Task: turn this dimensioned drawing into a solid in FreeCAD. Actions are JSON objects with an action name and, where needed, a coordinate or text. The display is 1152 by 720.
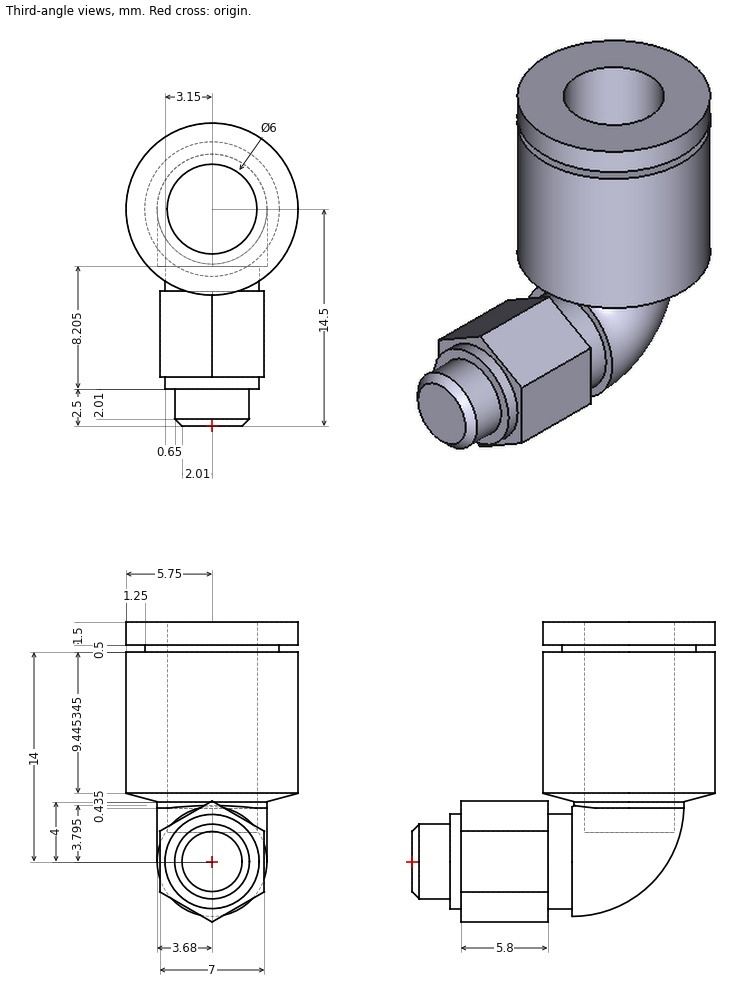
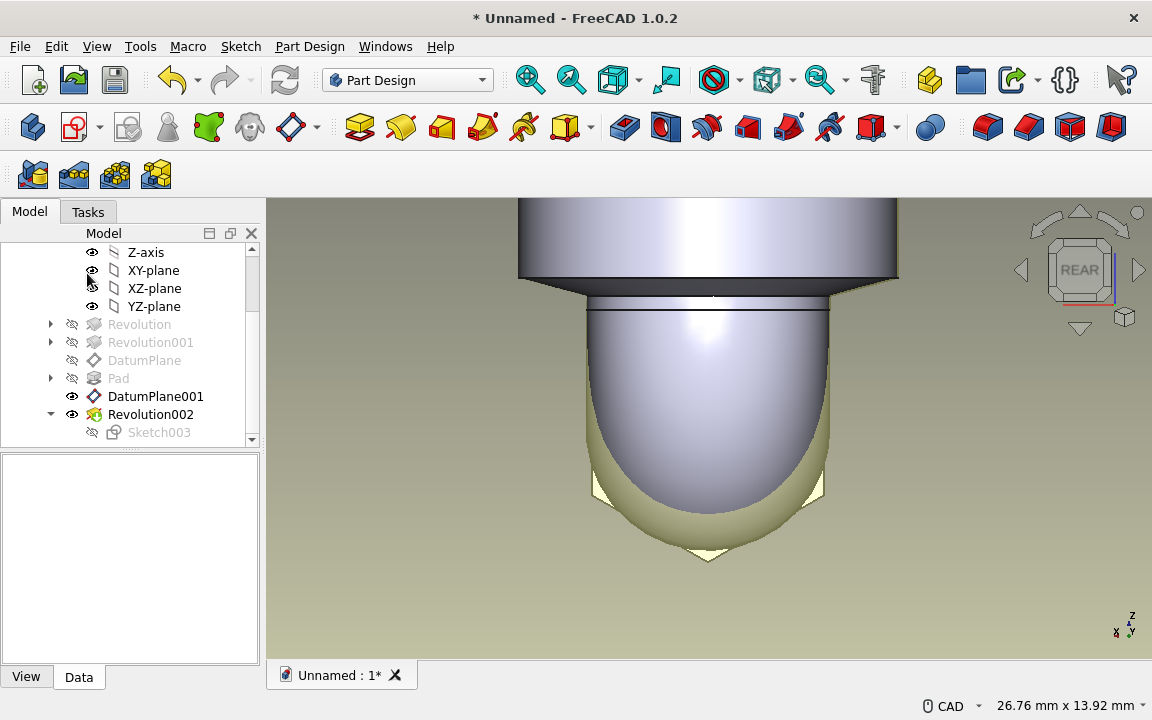
{"action": "left_click", "coordinate": [117, 396]}
{"action": "key", "text": "space"}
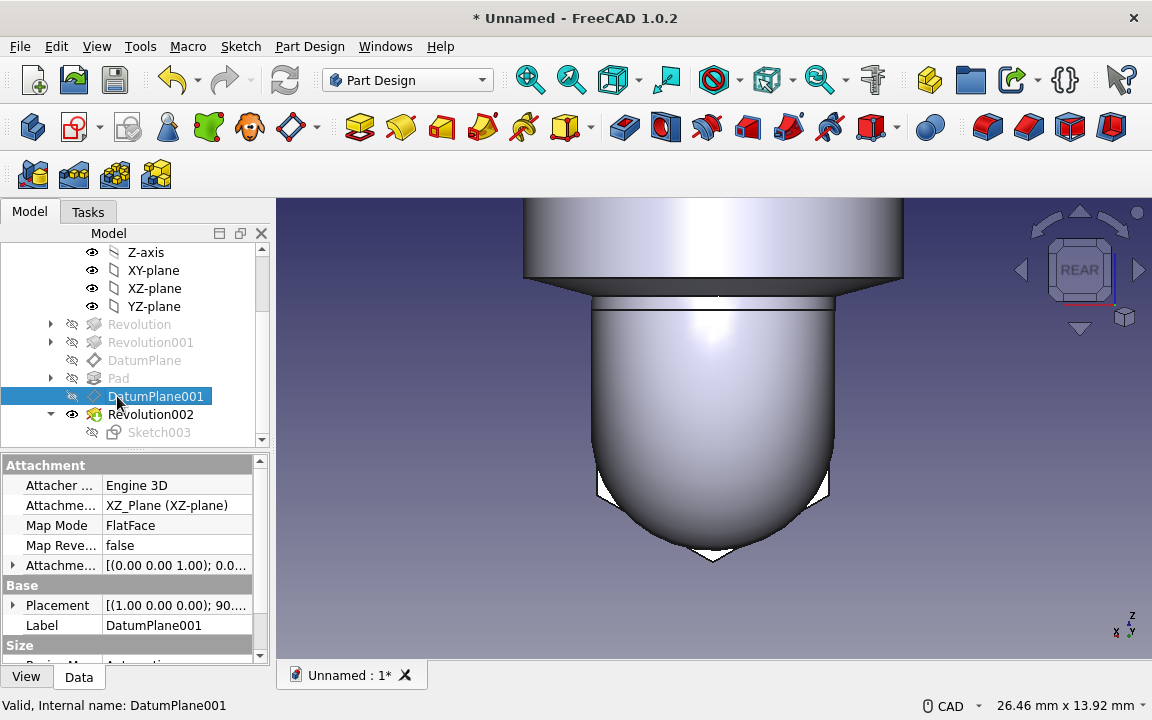
{"action": "left_click", "coordinate": [531, 80]}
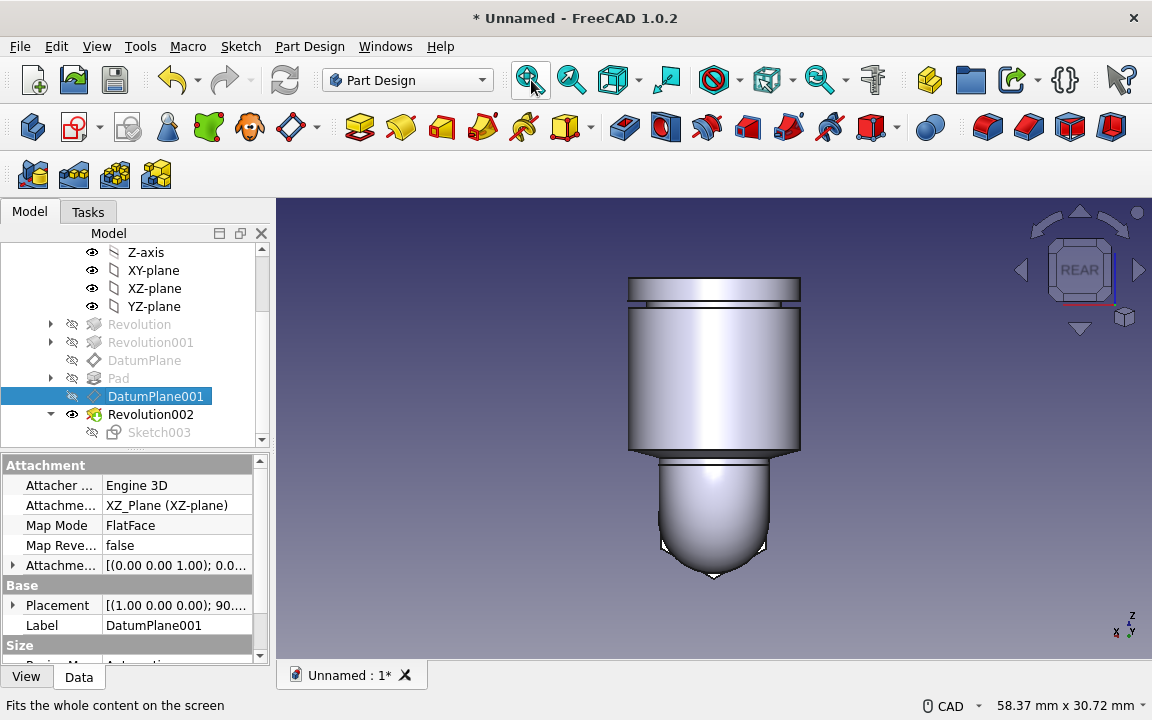
{"action": "key", "text": "0"}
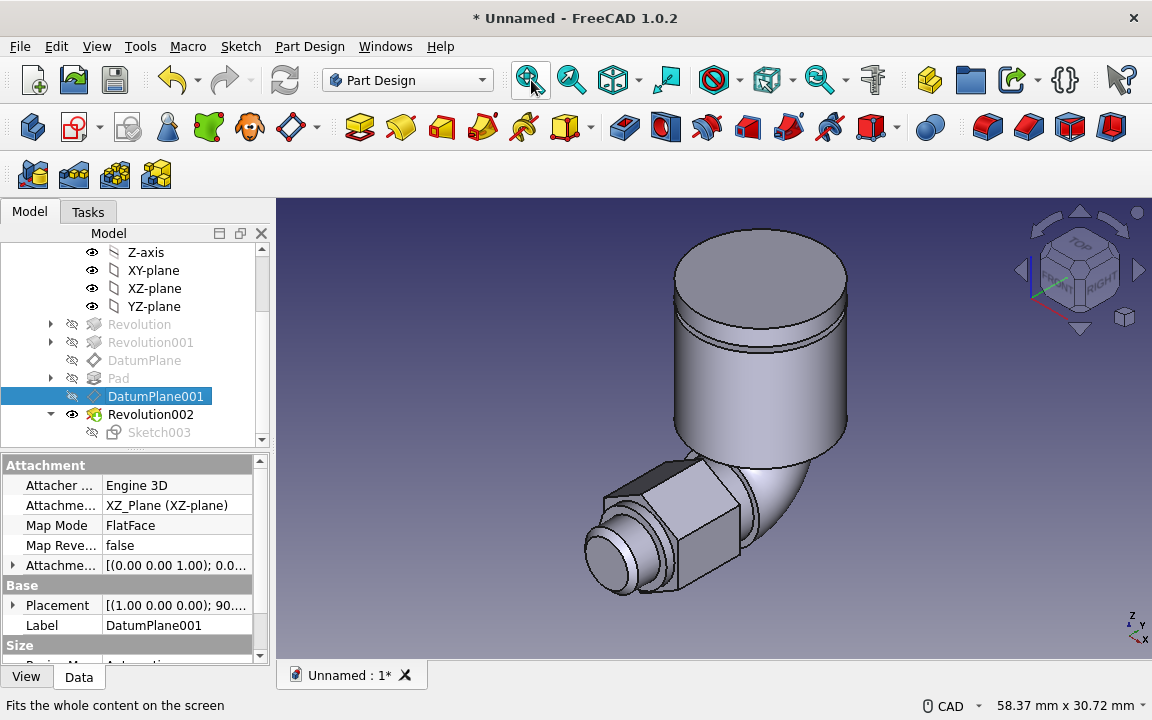
{"action": "left_click", "coordinate": [761, 278]}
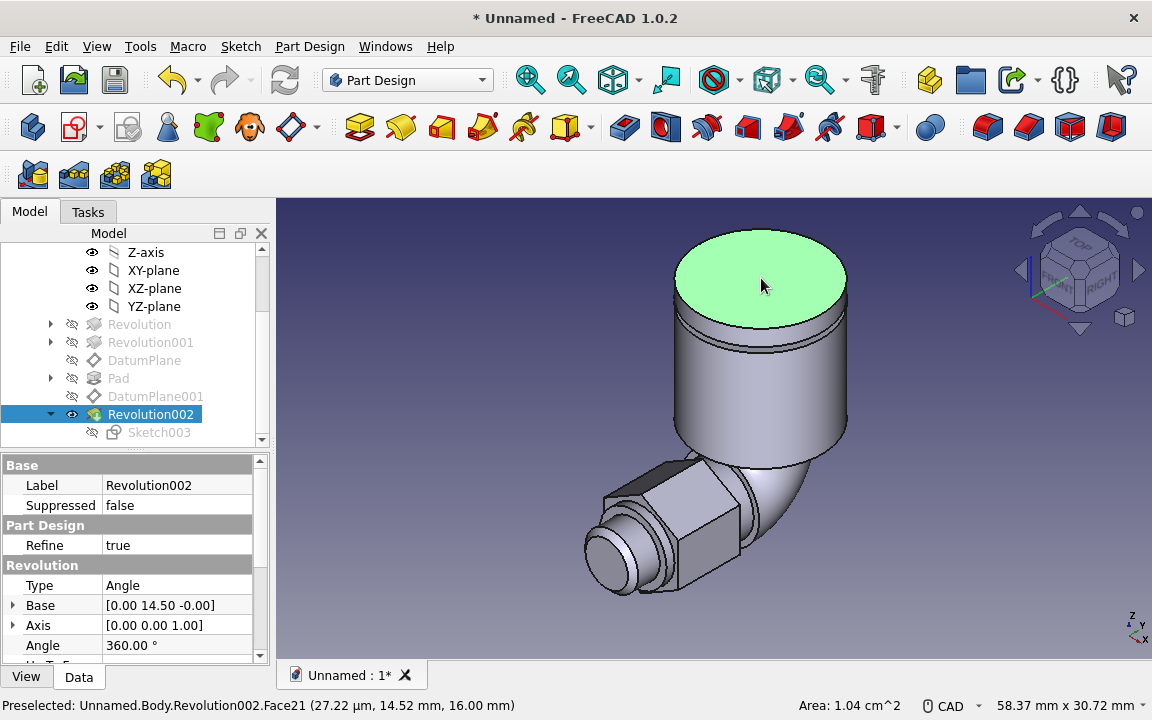
{"action": "left_click", "coordinate": [74, 128]}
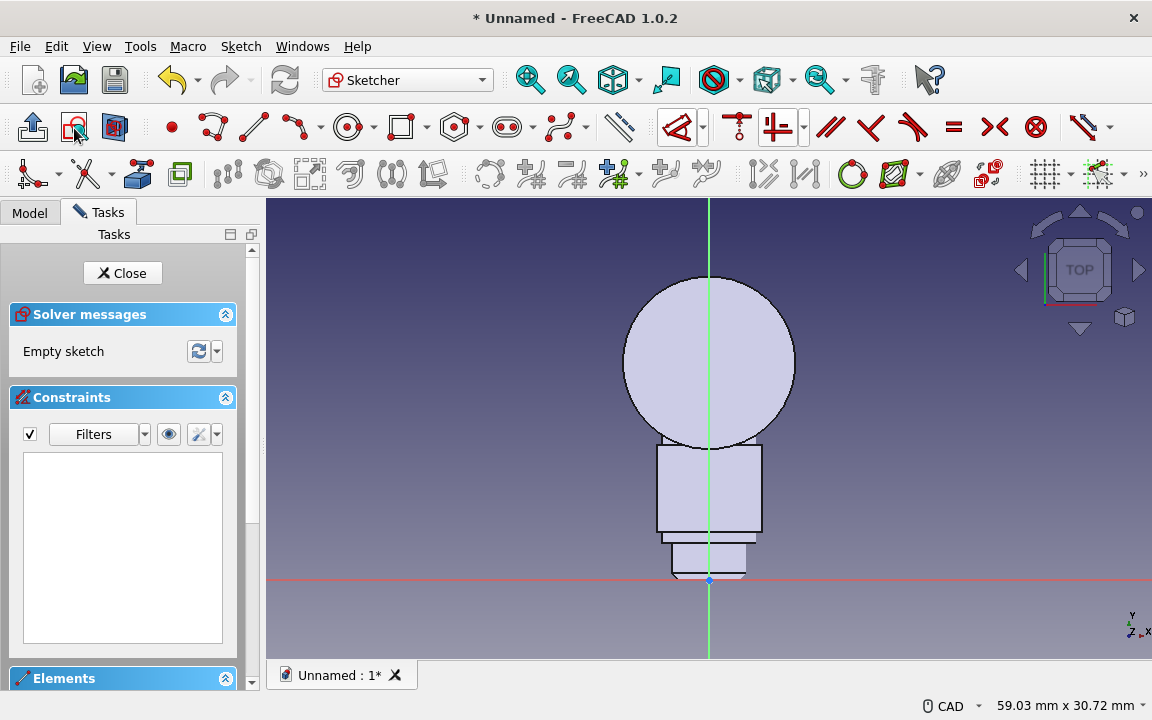
{"action": "scroll", "coordinate": [739, 334], "scroll_direction": "up", "scroll_amount": 6}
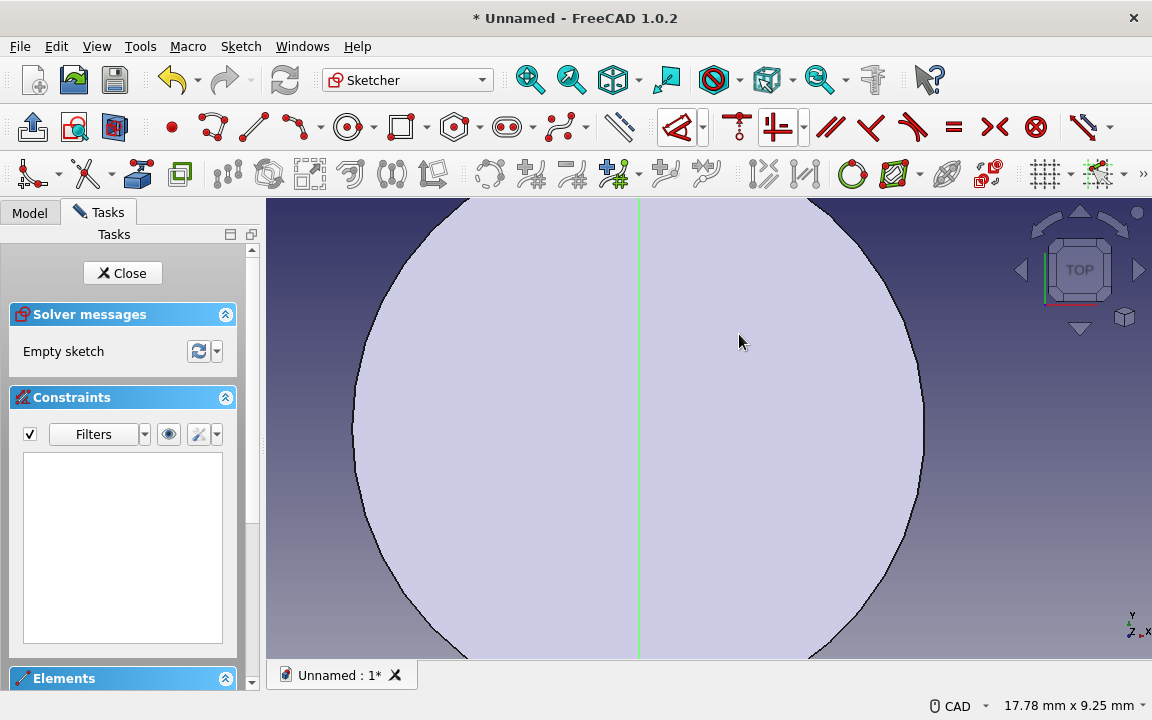
{"action": "left_click", "coordinate": [348, 128]}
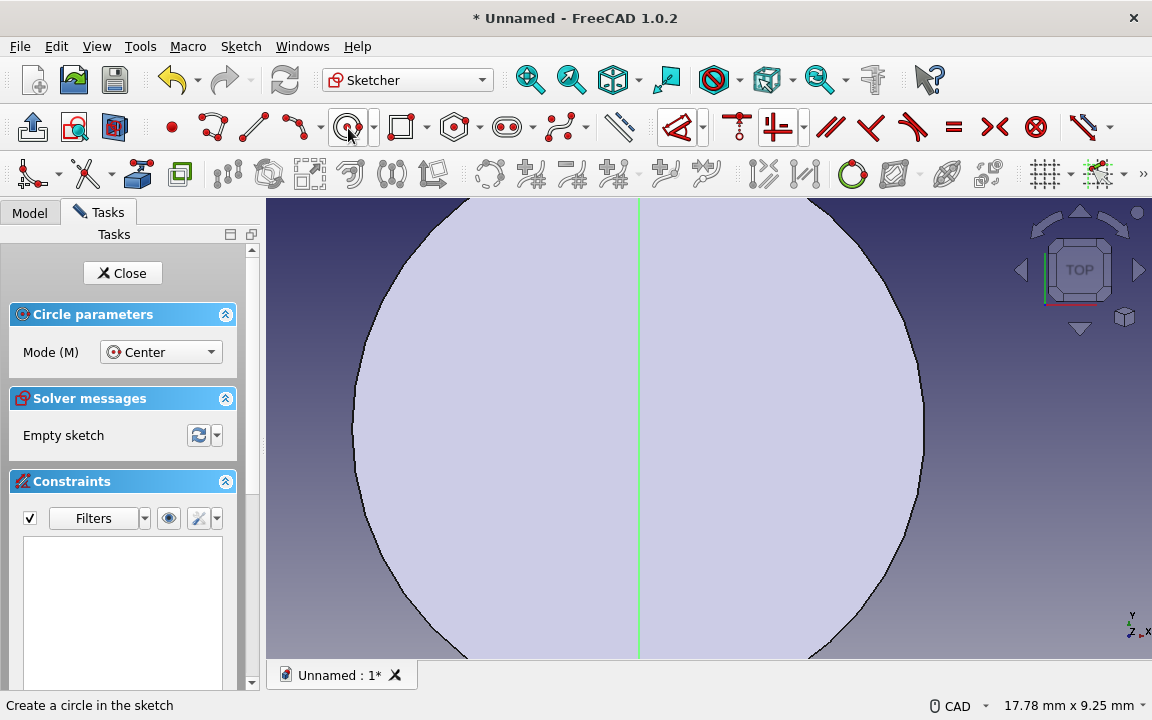
{"action": "left_click", "coordinate": [639, 429]}
{"action": "left_click", "coordinate": [744, 323]}
{"action": "key", "text": "Escape"}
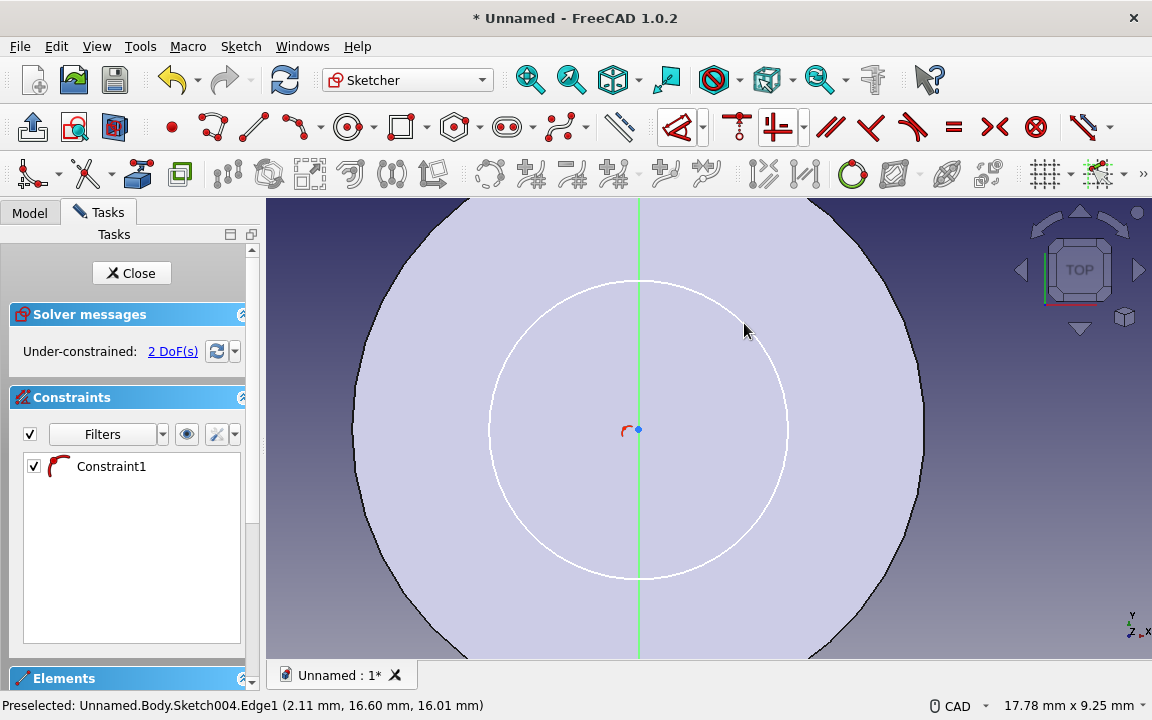
{"action": "left_click", "coordinate": [744, 324]}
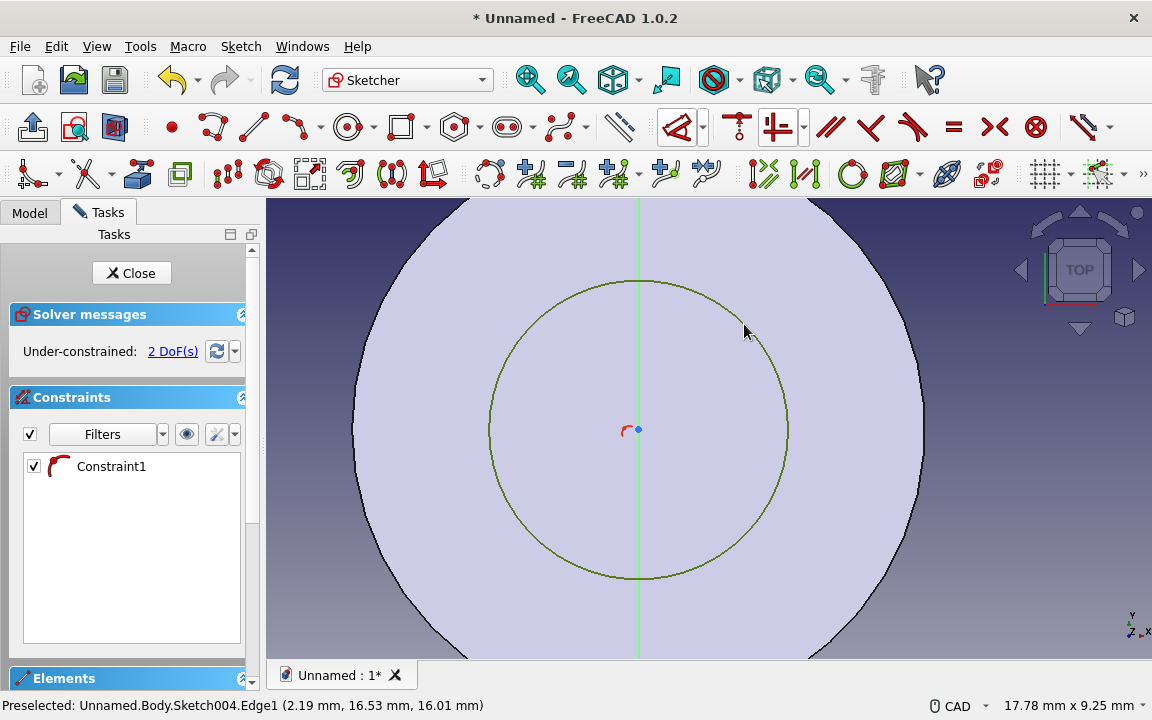
{"action": "key", "text": "k o"}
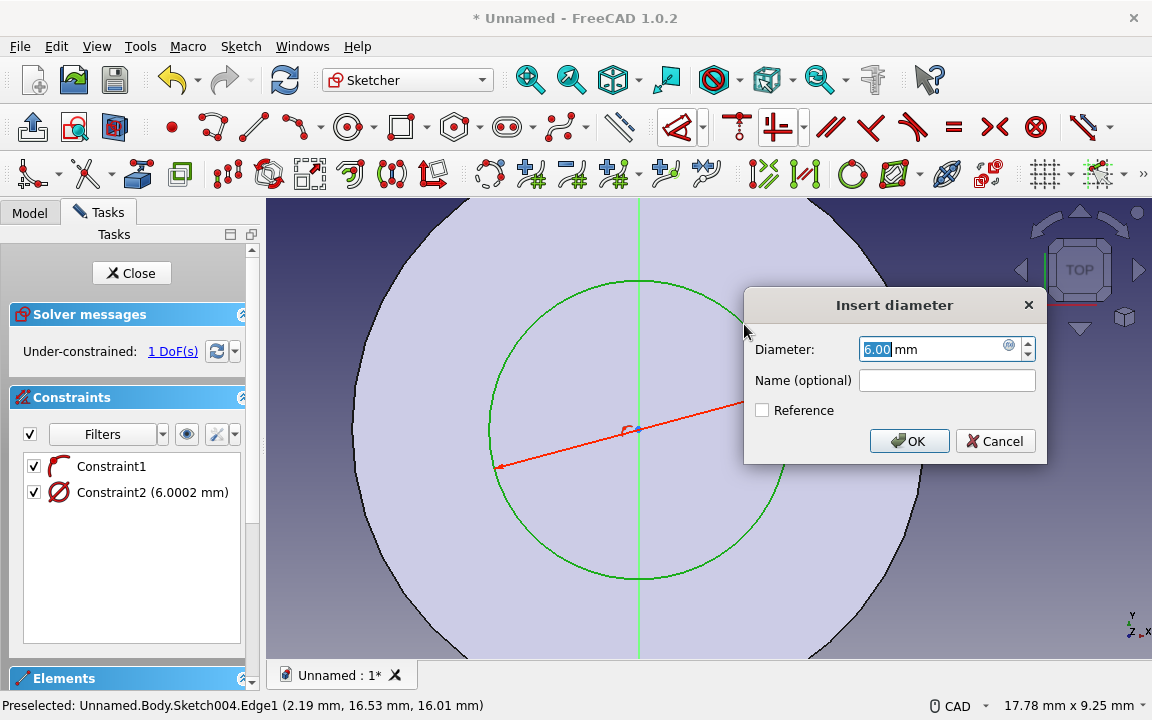
{"action": "type", "text": "6"}
{"action": "key", "text": "Return"}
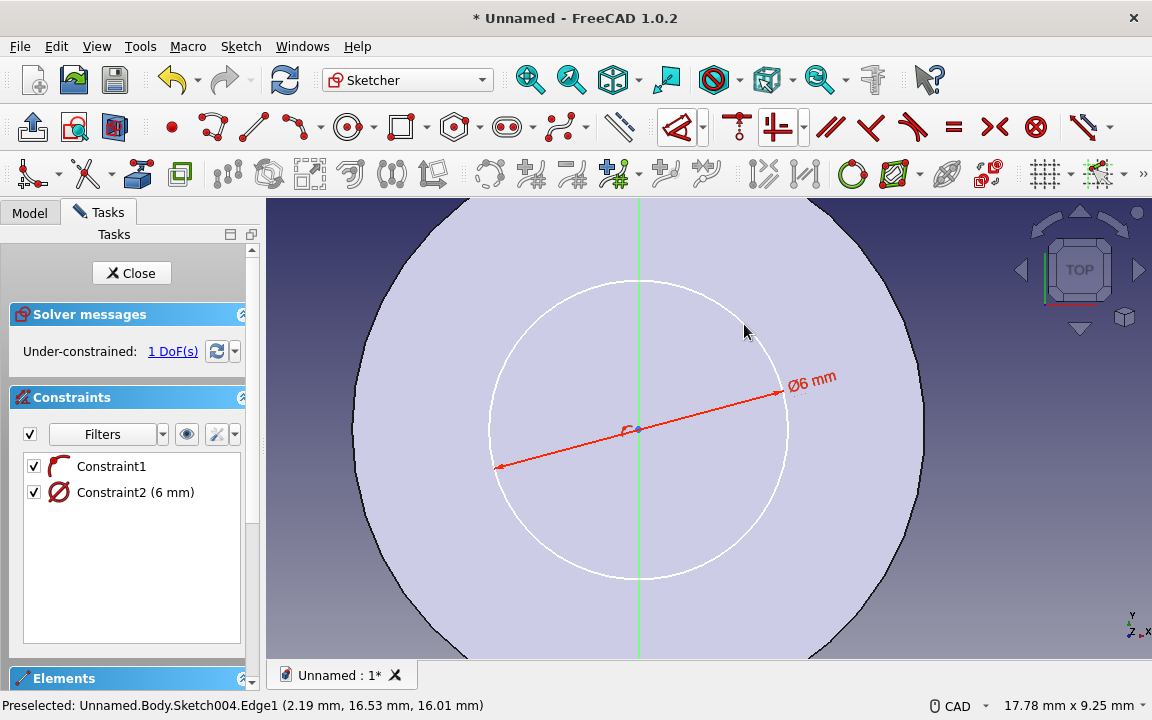
{"action": "left_click", "coordinate": [639, 430]}